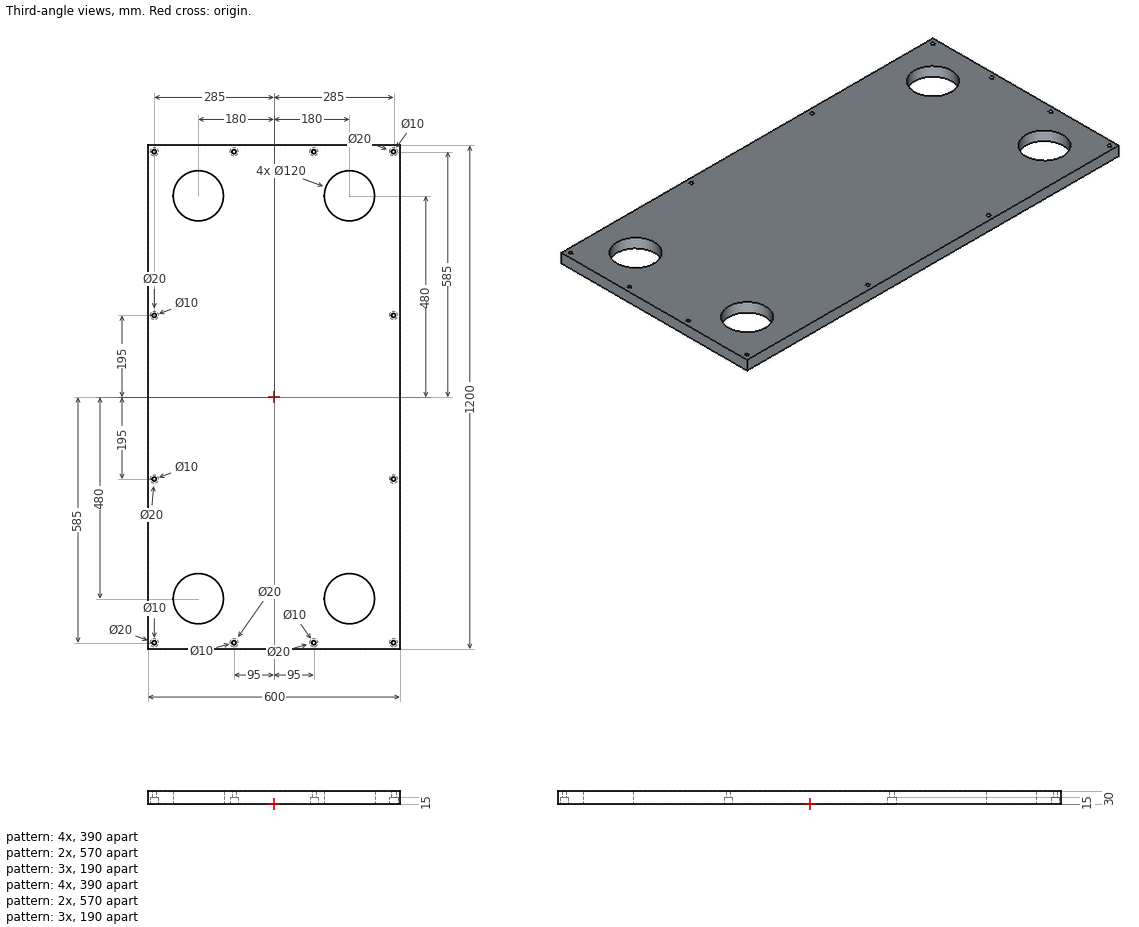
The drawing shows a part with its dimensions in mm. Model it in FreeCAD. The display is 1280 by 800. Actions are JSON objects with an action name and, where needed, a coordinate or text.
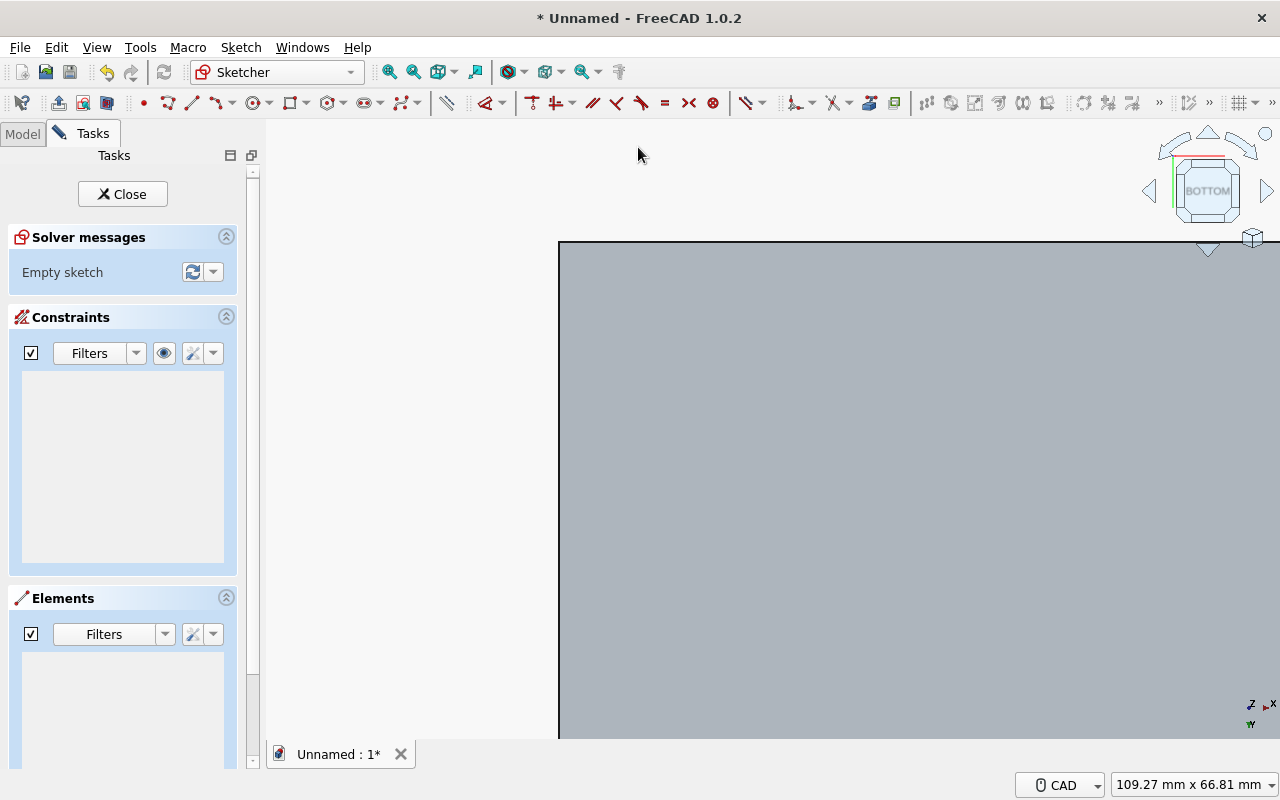
{"action": "scroll", "coordinate": [696, 366], "scroll_direction": "up", "scroll_amount": 7}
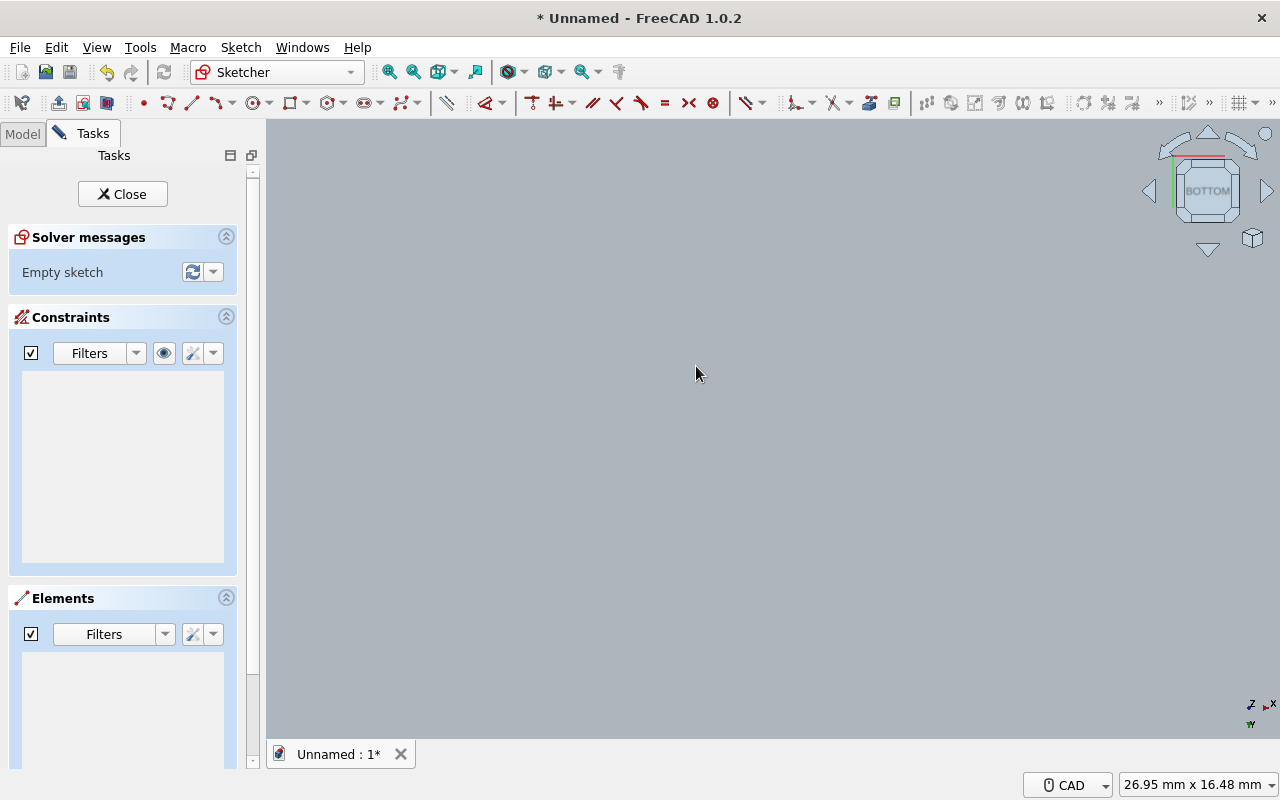
{"action": "left_click", "coordinate": [254, 104]}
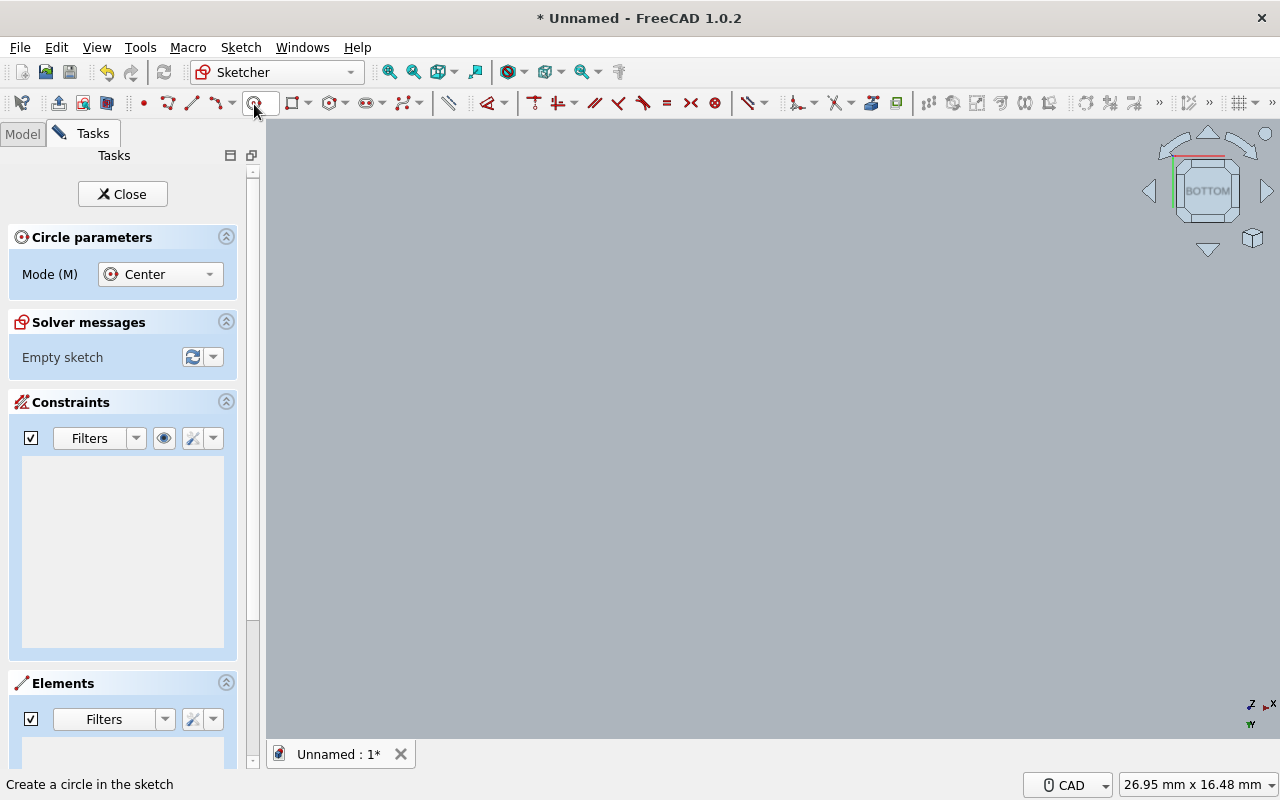
{"action": "left_click", "coordinate": [702, 428]}
{"action": "mouse_move", "coordinate": [835, 295]}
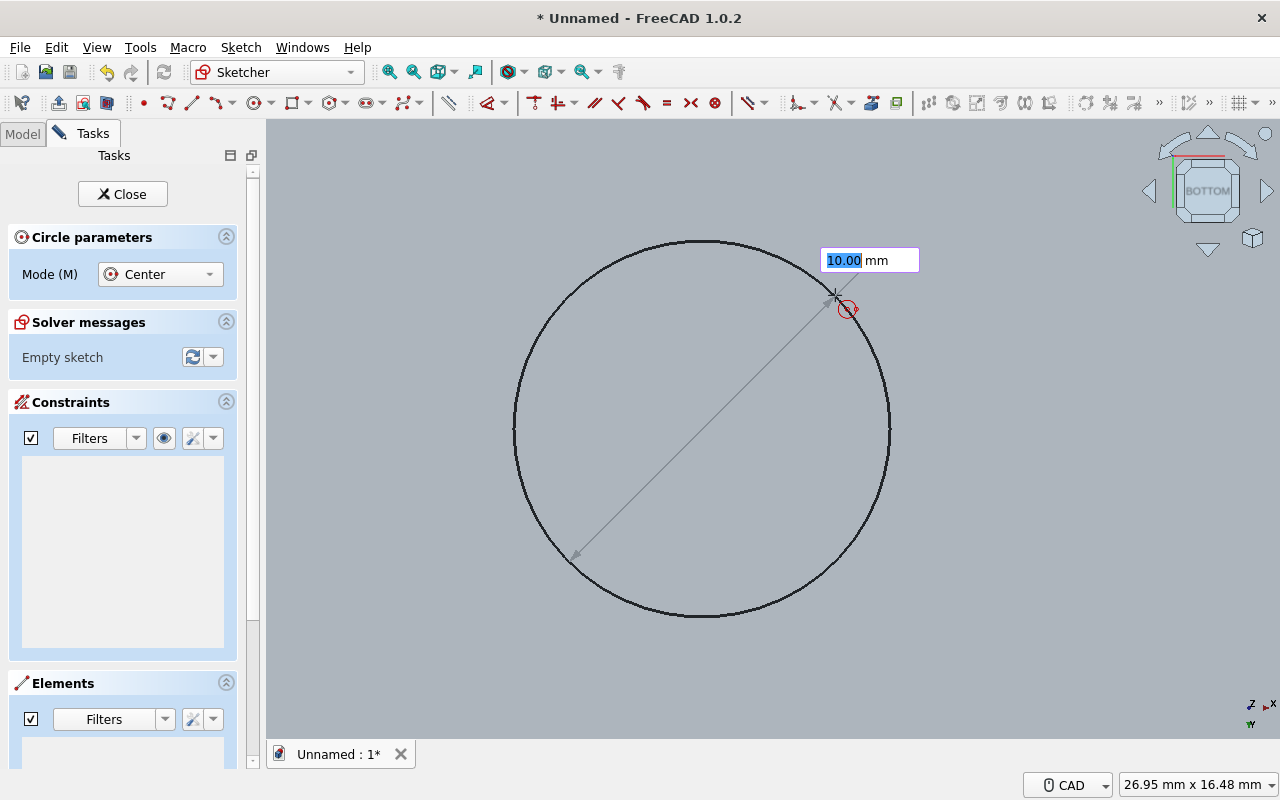
{"action": "type", "text": "10"}
{"action": "key", "text": "Return"}
{"action": "key", "text": "Escape"}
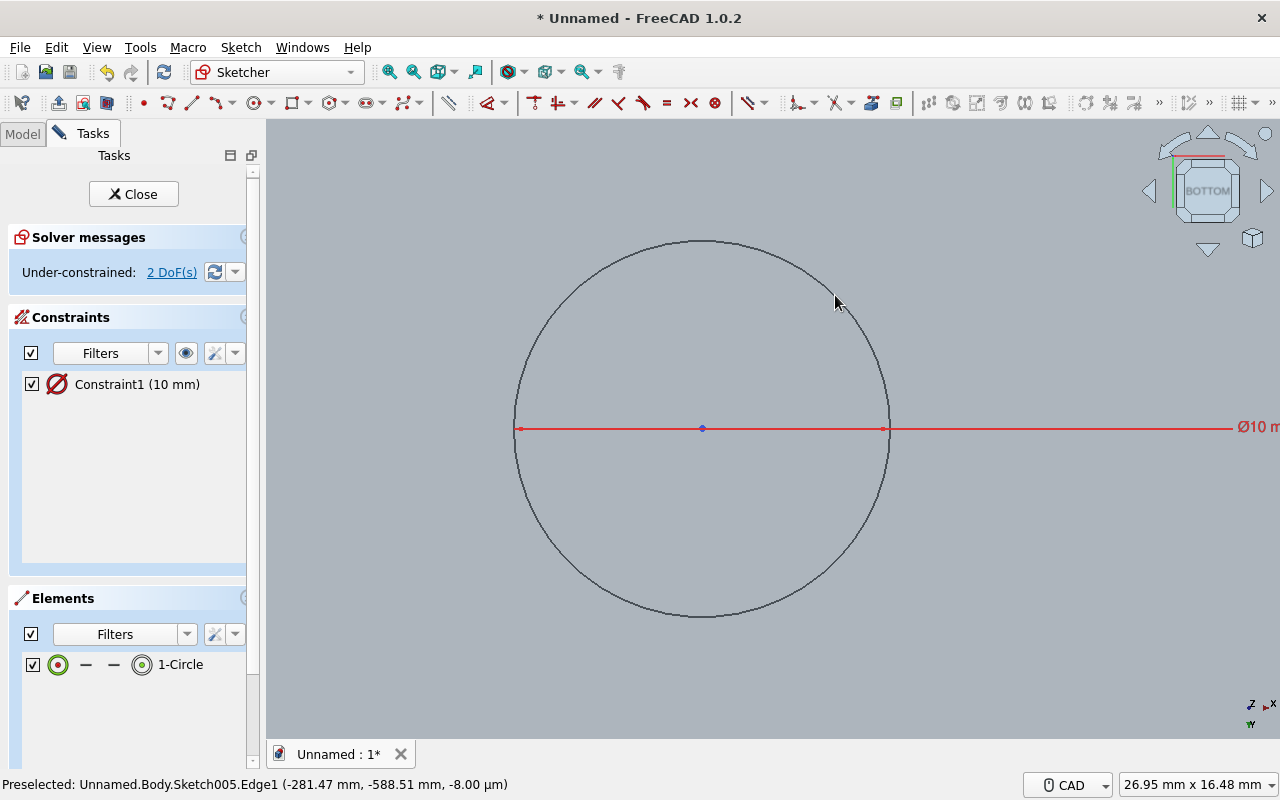
{"action": "left_click", "coordinate": [488, 104]}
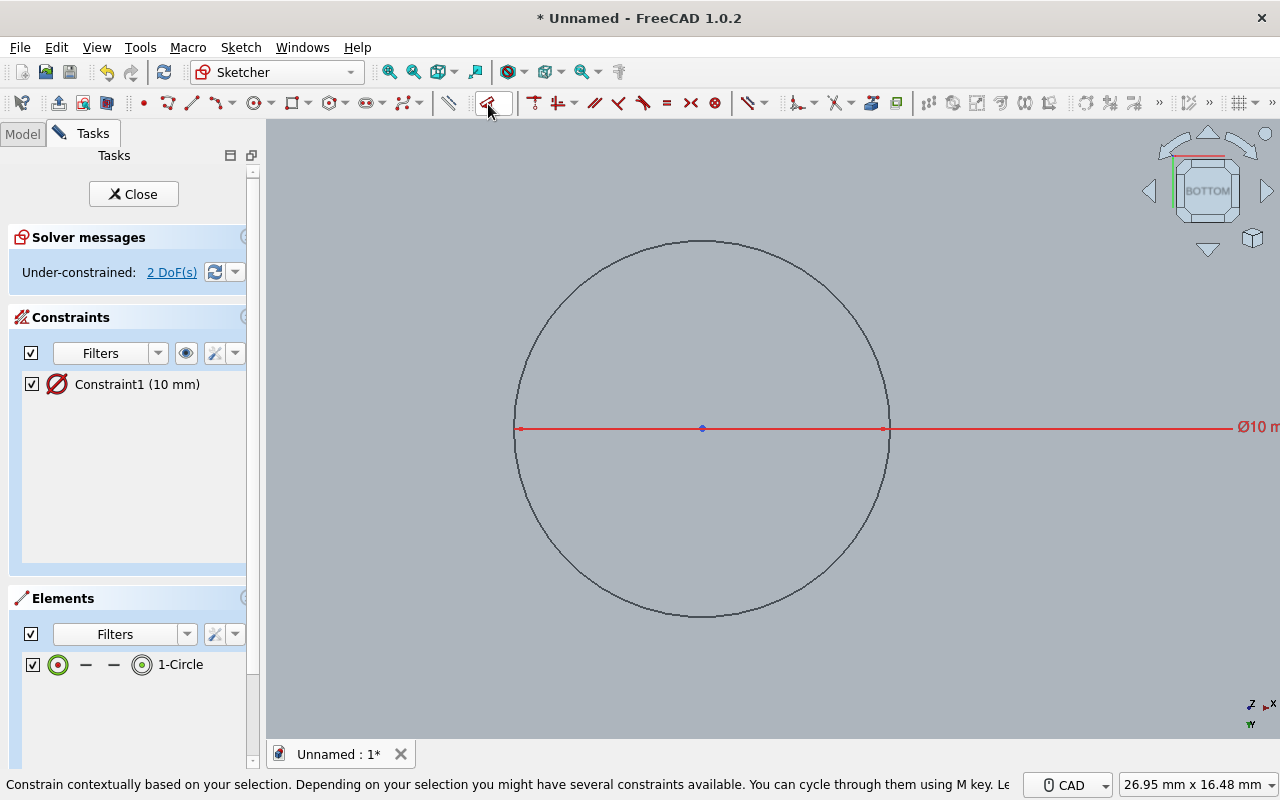
{"action": "left_click", "coordinate": [702, 429]}
{"action": "left_click", "coordinate": [909, 395]}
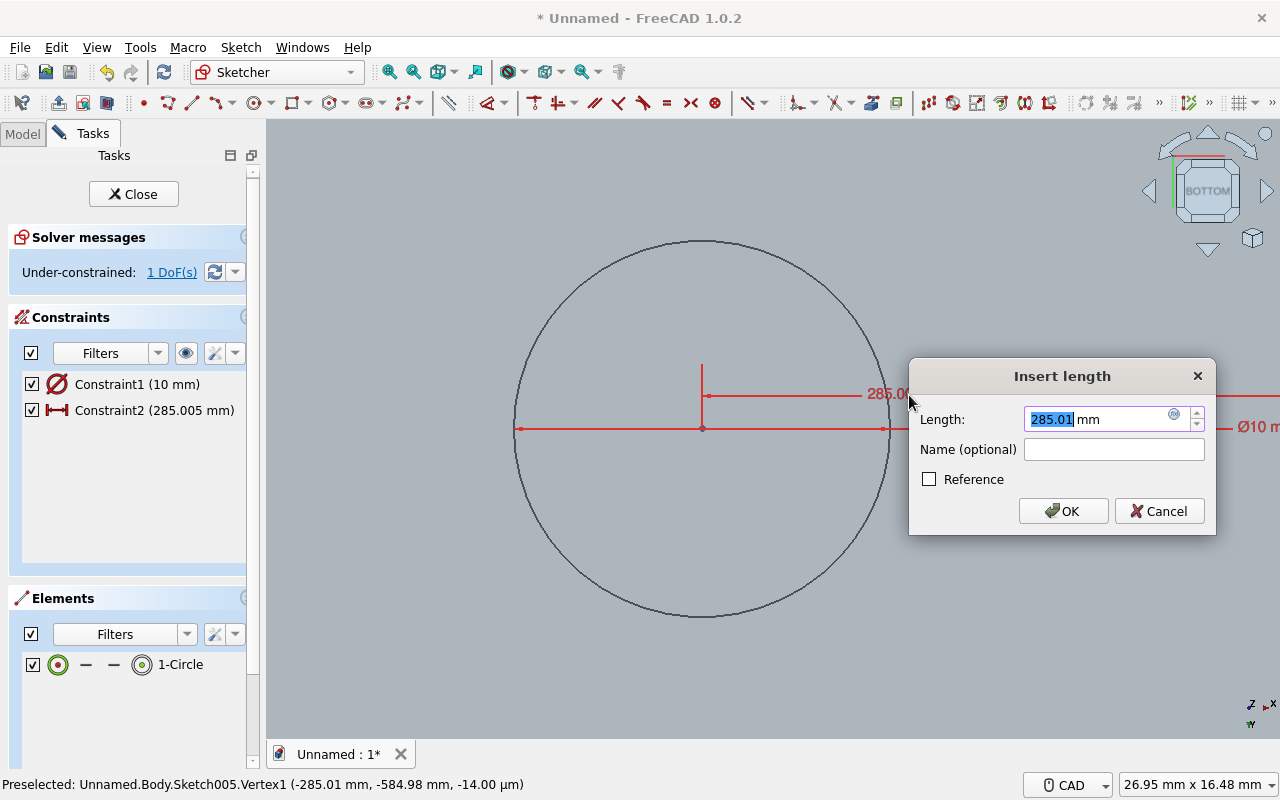
{"action": "type", "text": "285"}
{"action": "key", "text": "Return"}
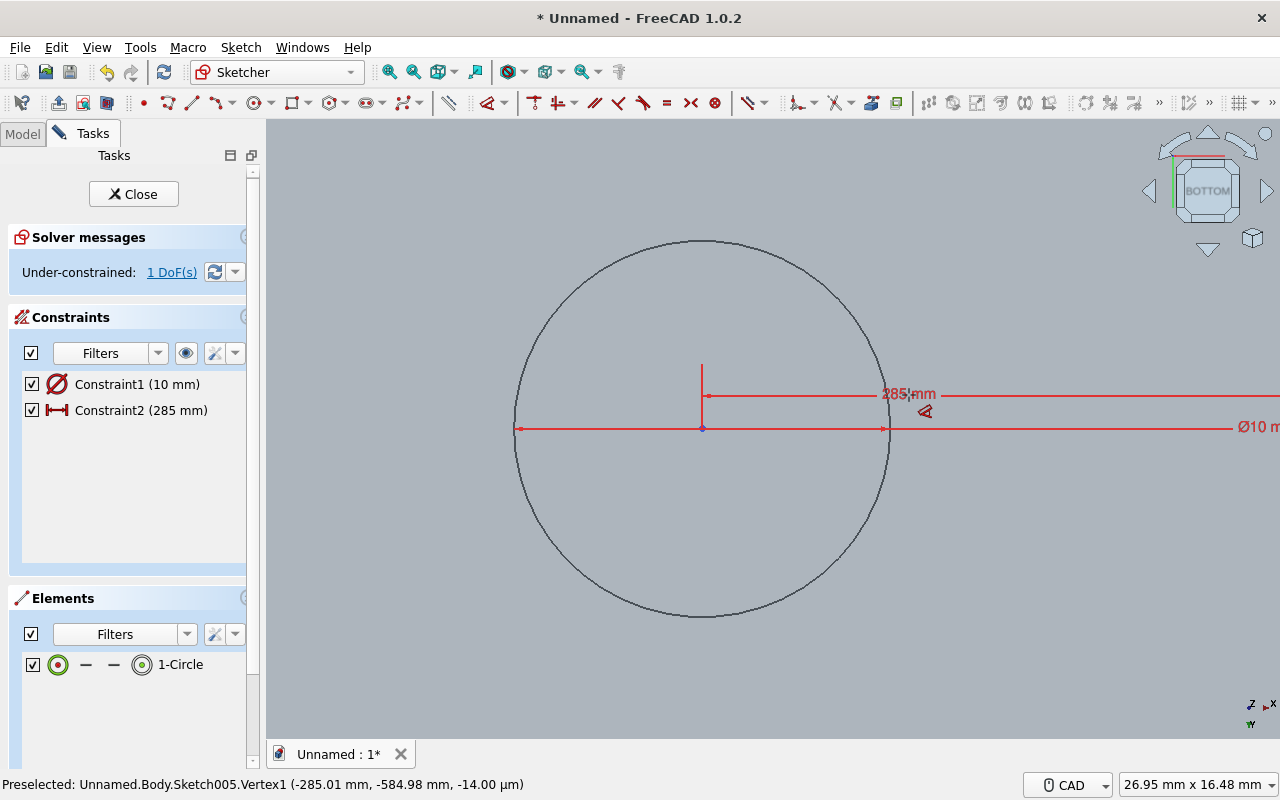
{"action": "left_click", "coordinate": [702, 429]}
{"action": "left_click", "coordinate": [668, 570]}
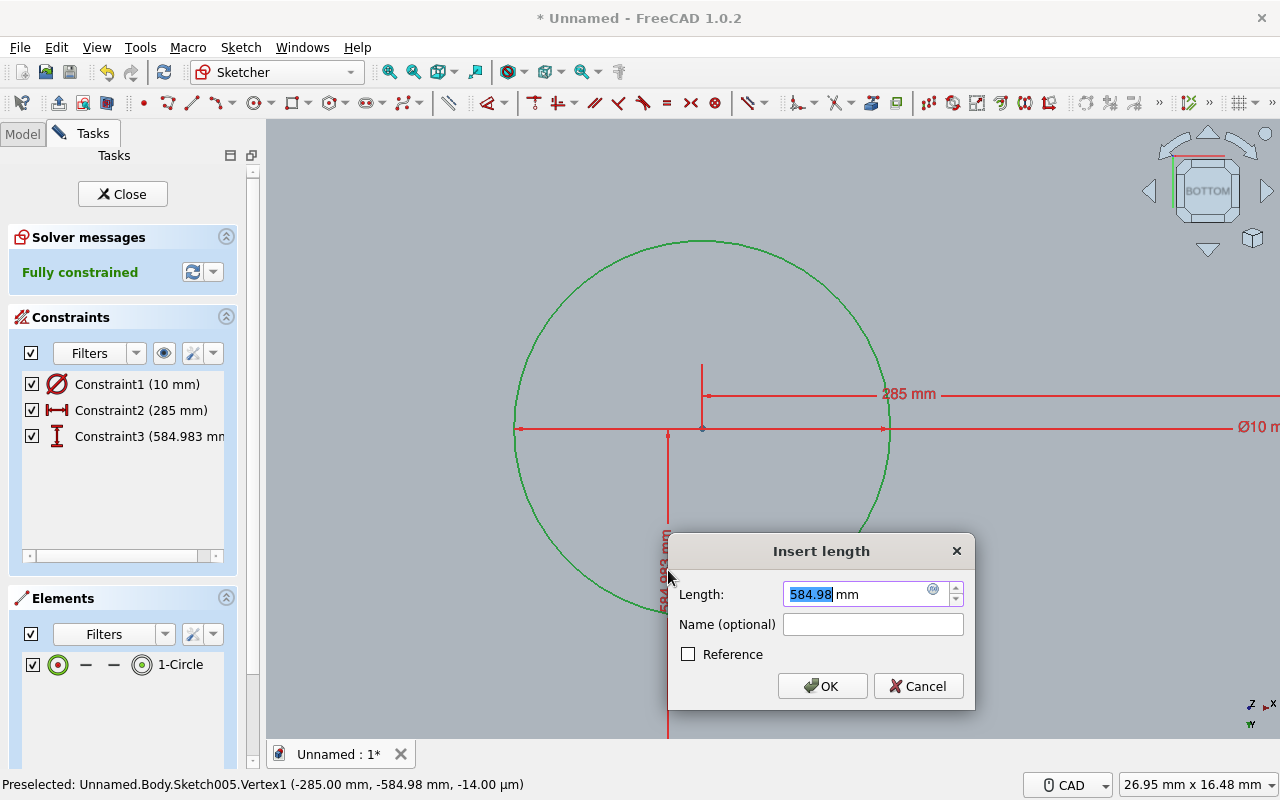
{"action": "type", "text": "585"}
{"action": "key", "text": "Return"}
{"action": "key", "text": "Escape"}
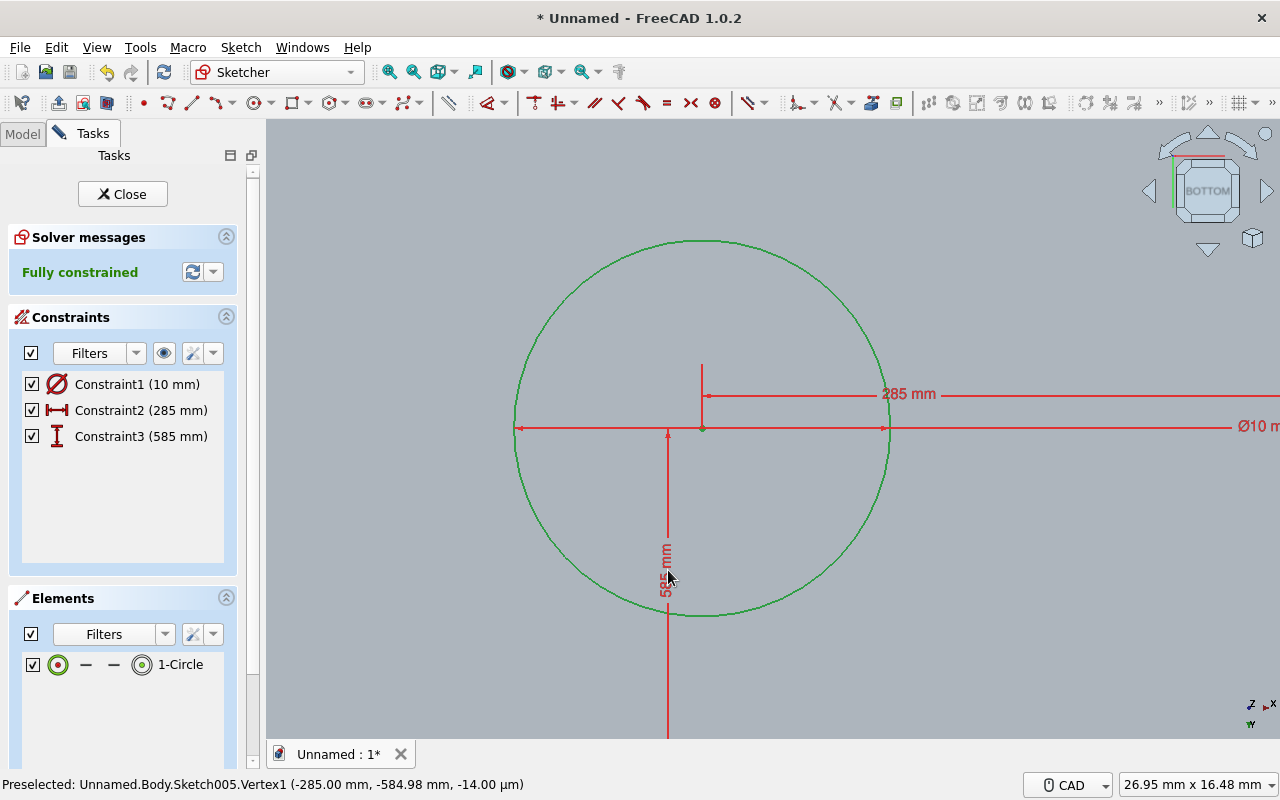
{"action": "left_click", "coordinate": [123, 194]}